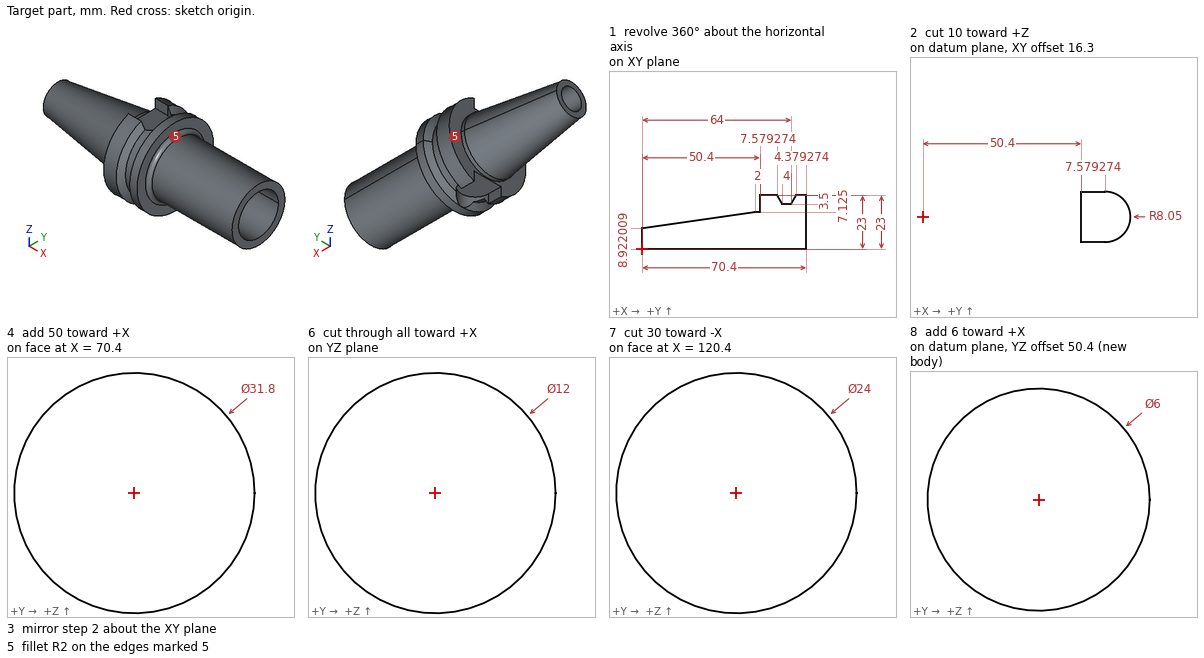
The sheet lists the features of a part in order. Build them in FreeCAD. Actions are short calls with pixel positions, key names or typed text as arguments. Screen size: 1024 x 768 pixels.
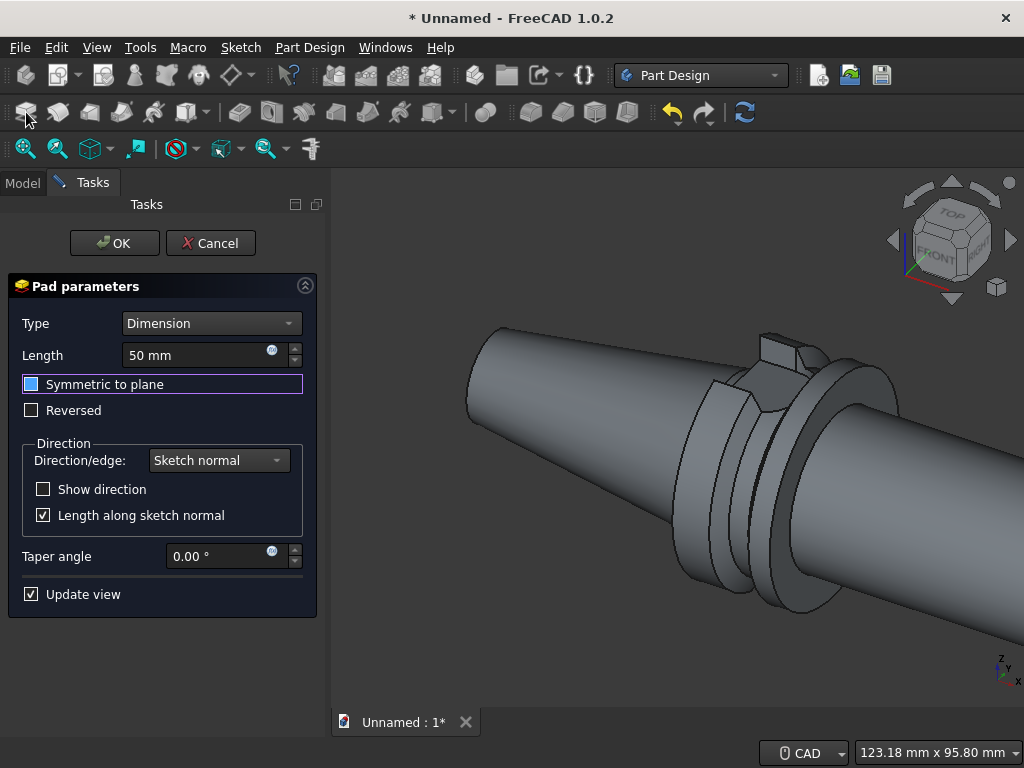
click(115, 243)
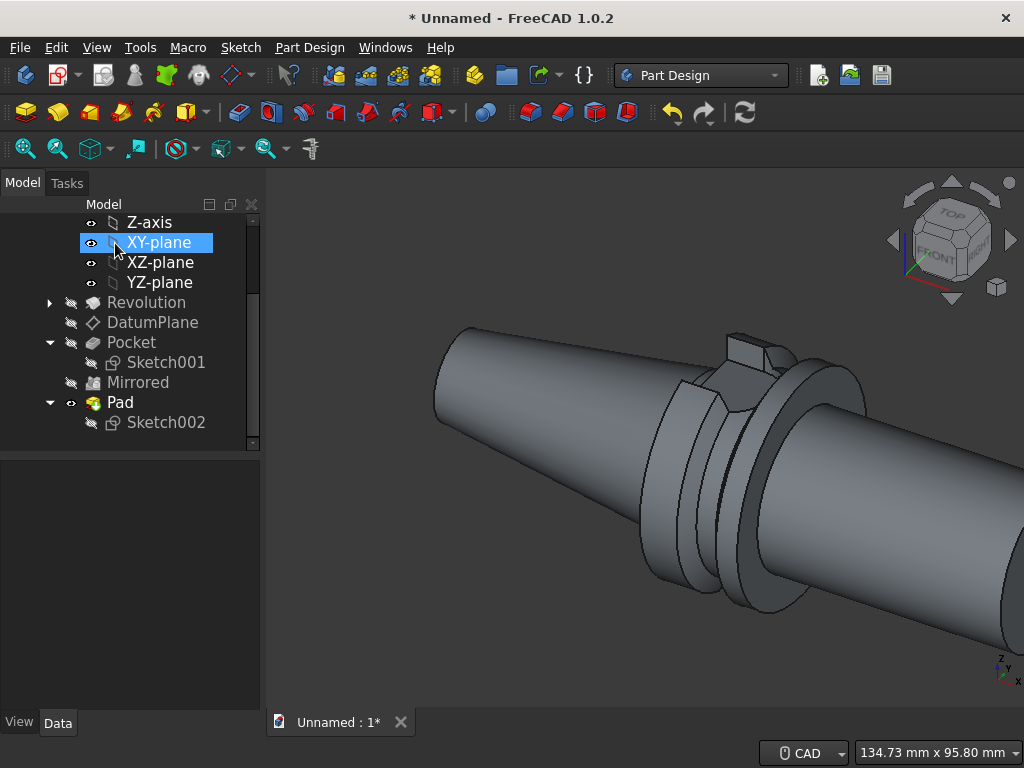
click(26, 150)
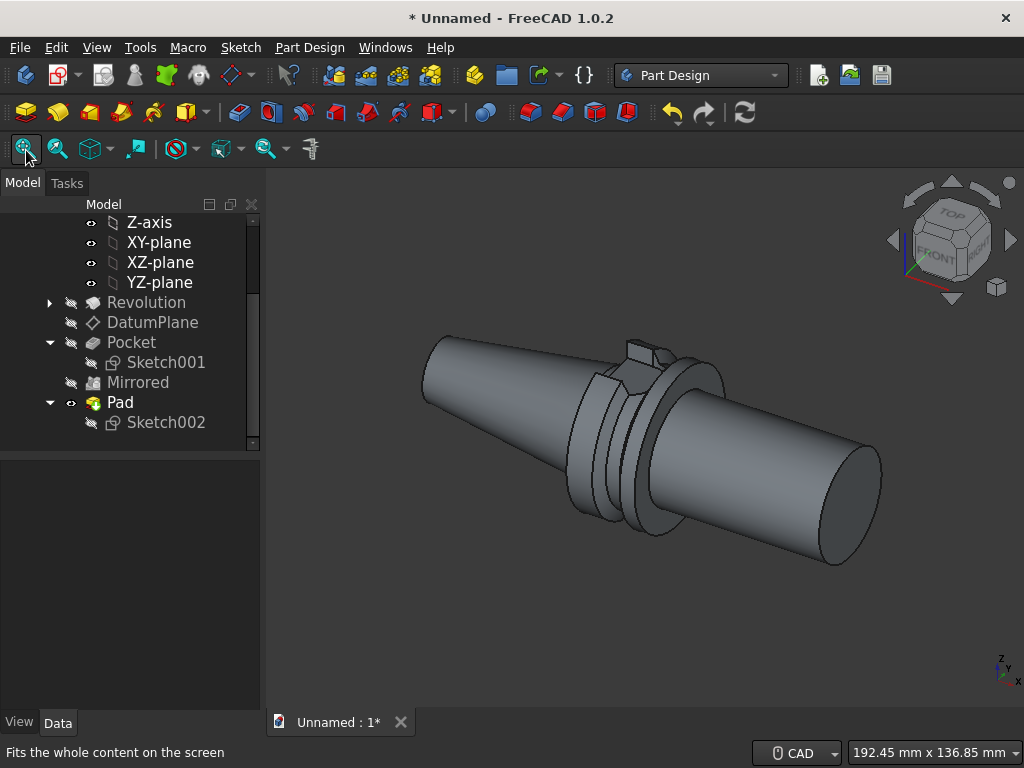
key(0)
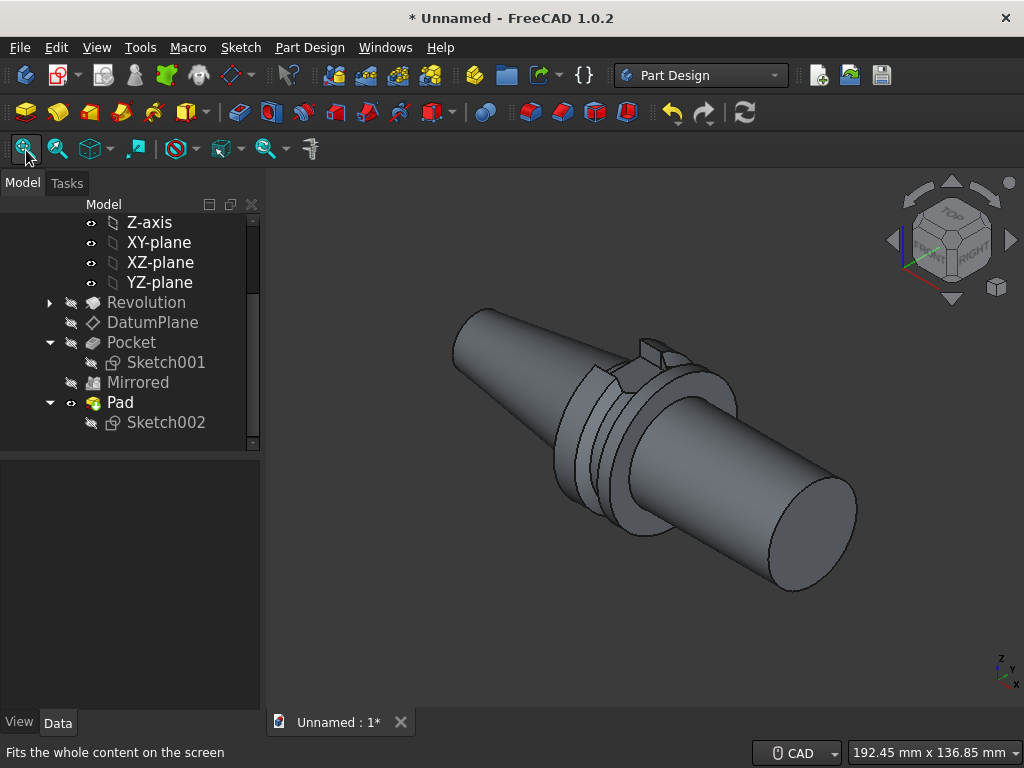
key(2)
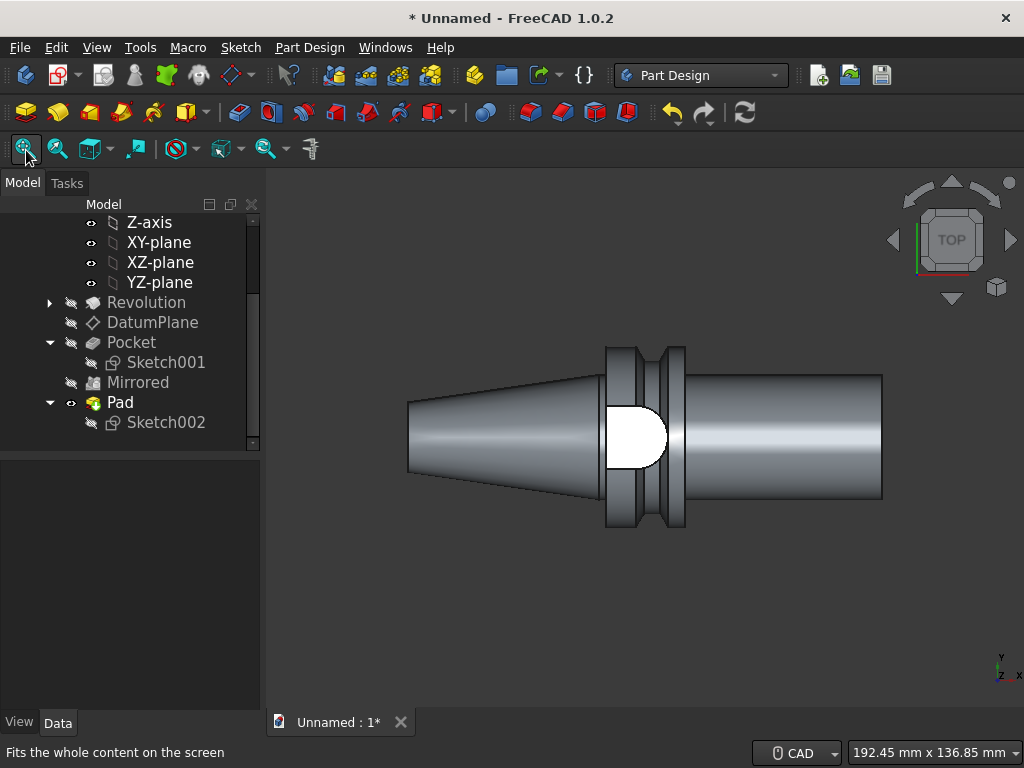
key(1)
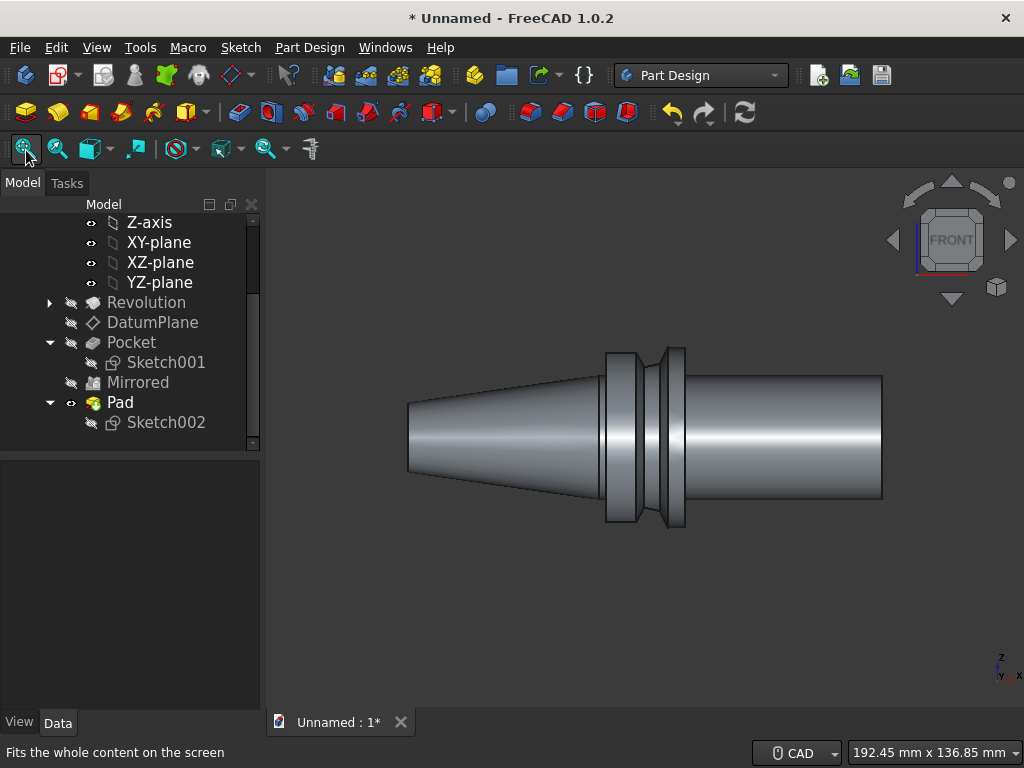
key(3)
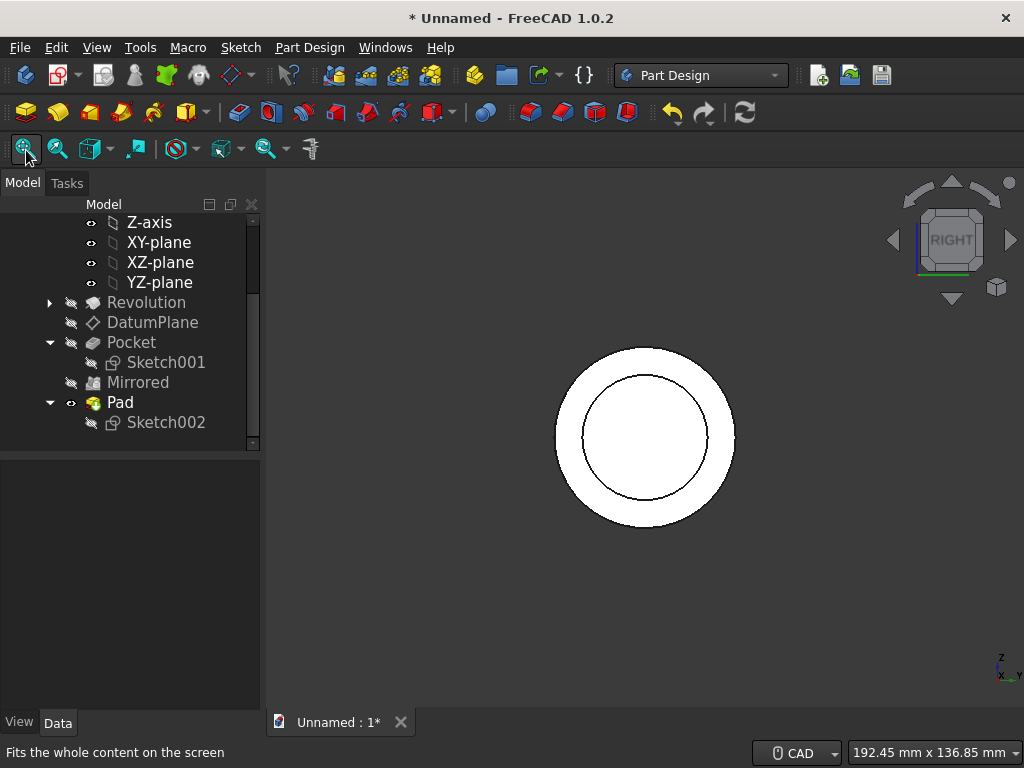
key(v)
key(f)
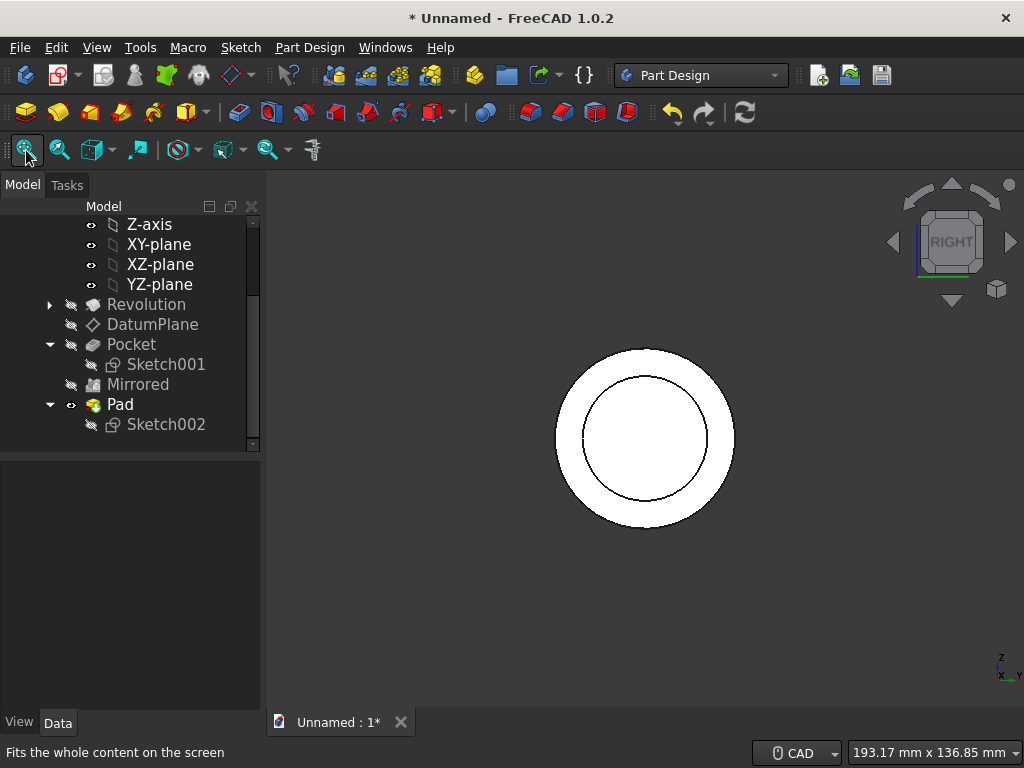
key(5)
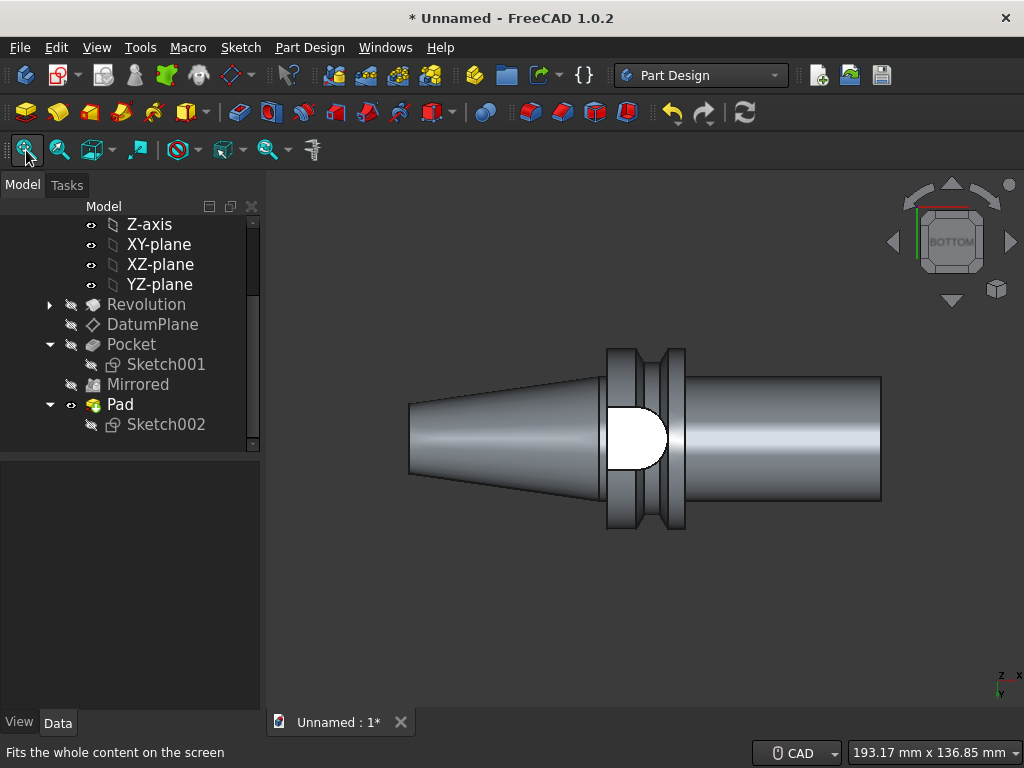
key(4)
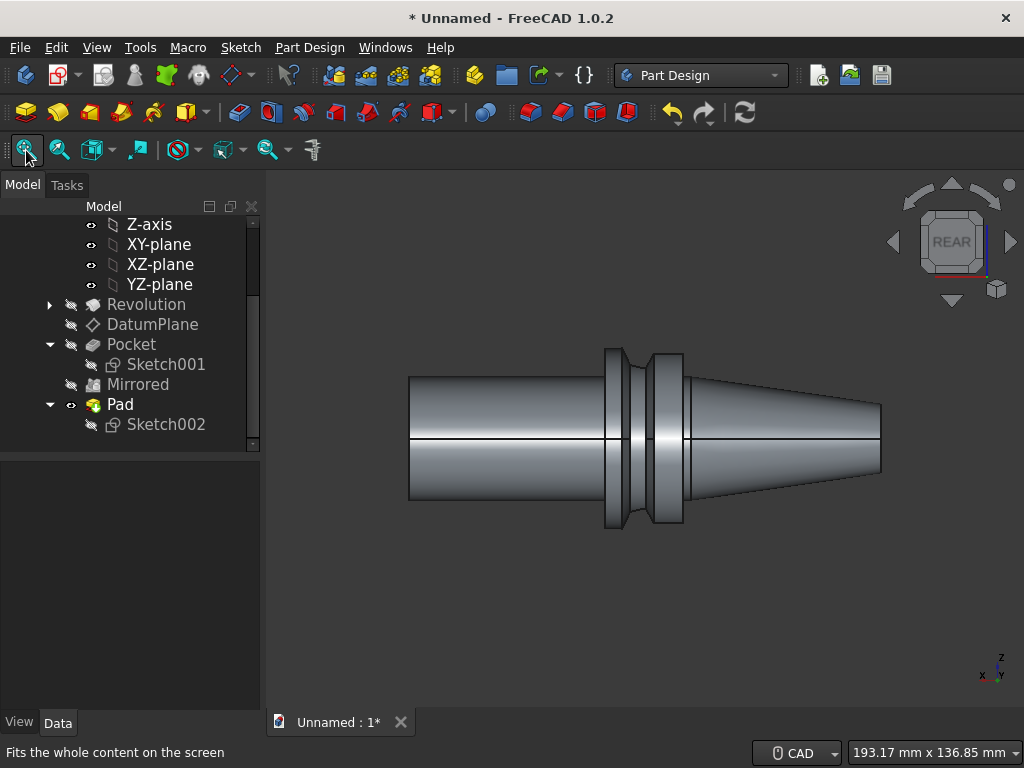
key(6)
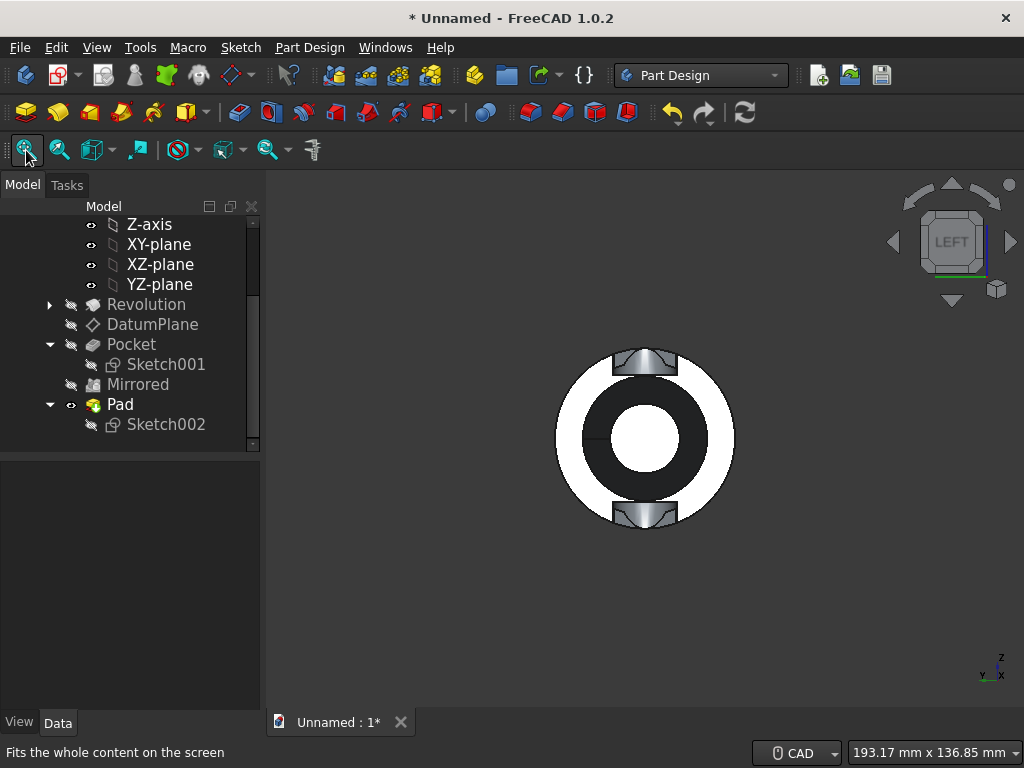
click(28, 150)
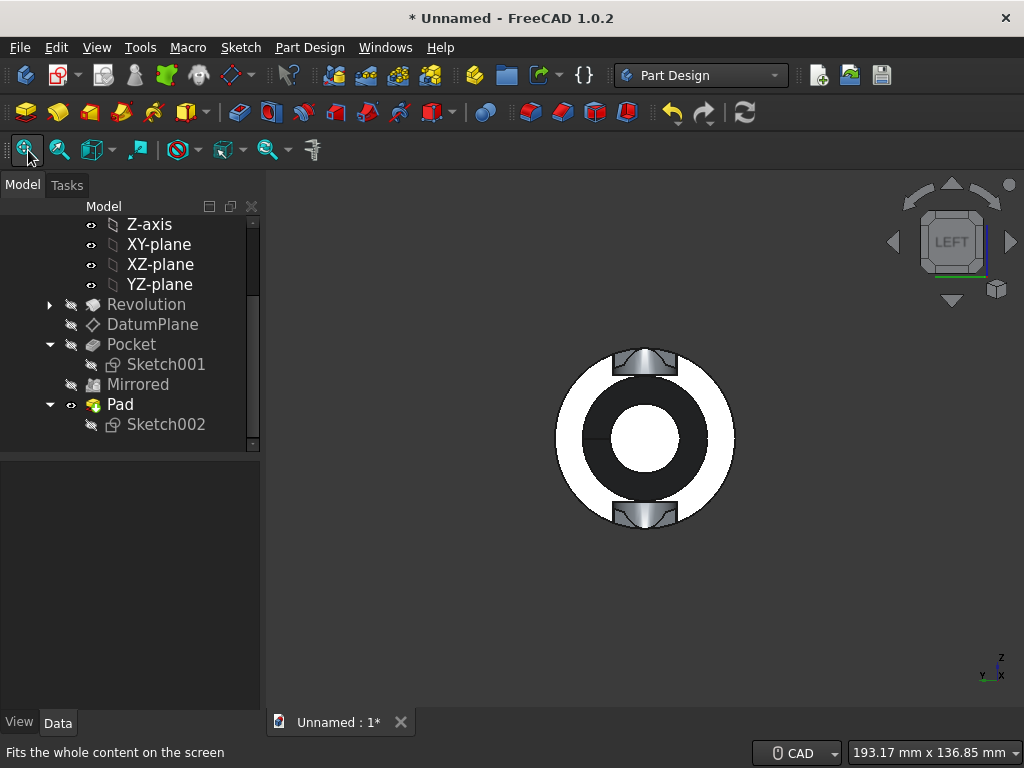
key(v)
key(3)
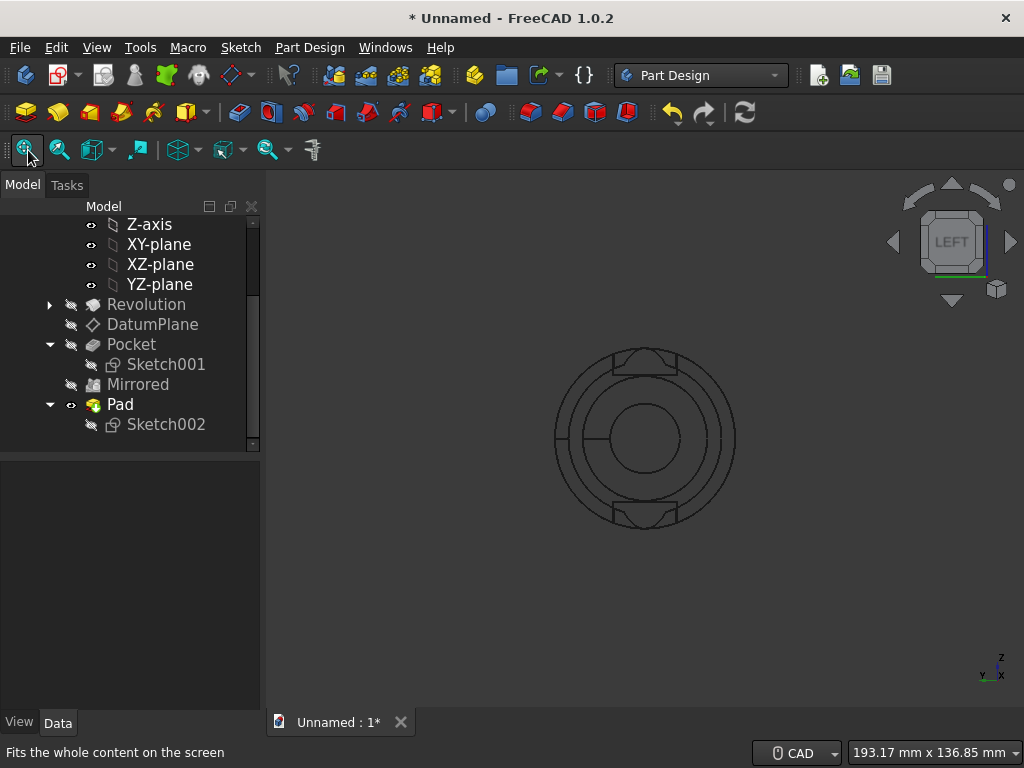
key(0)